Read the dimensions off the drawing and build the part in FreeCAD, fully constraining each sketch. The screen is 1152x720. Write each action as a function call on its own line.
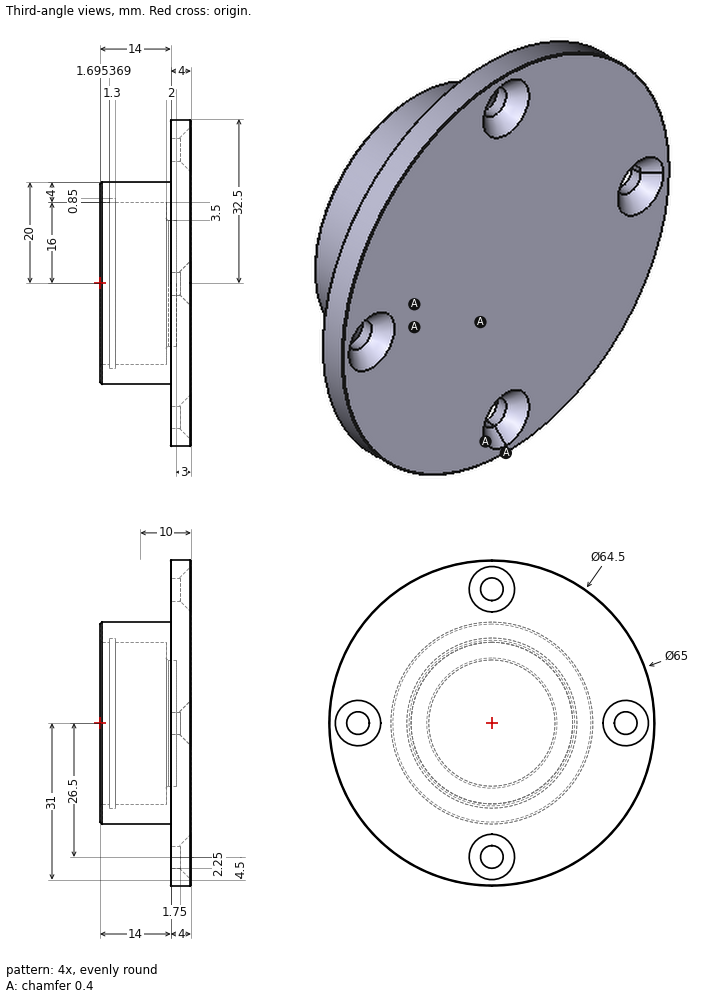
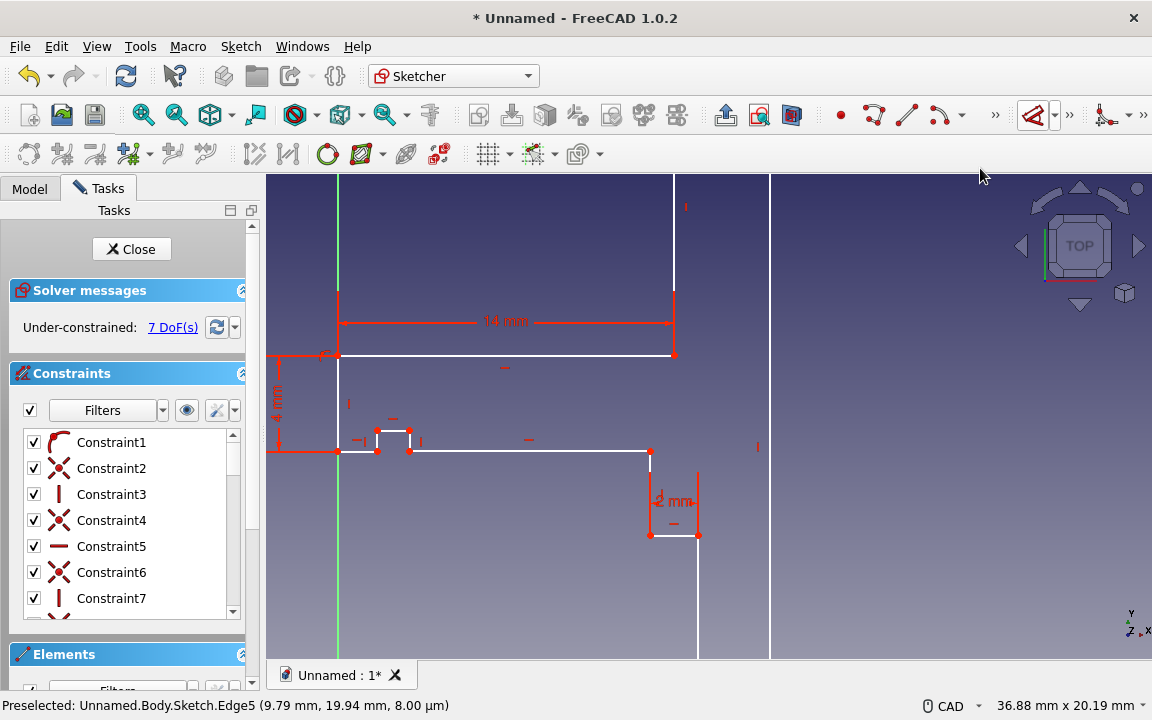
scroll(387, 431, up, 2)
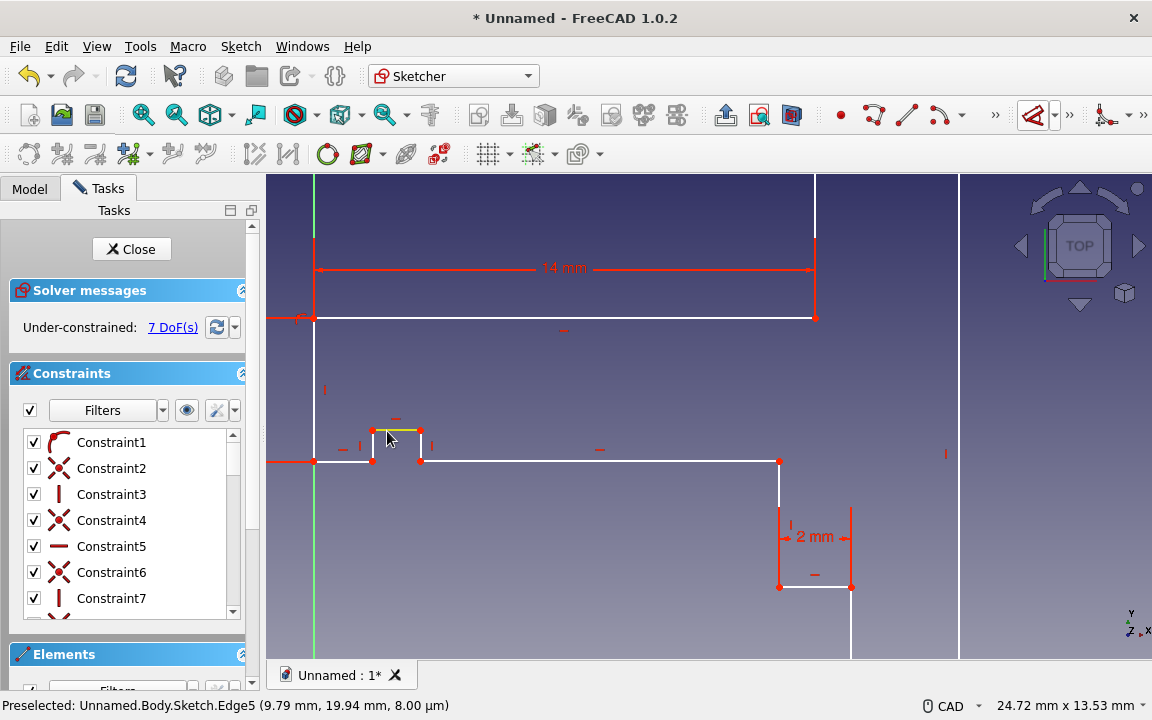
click(387, 430)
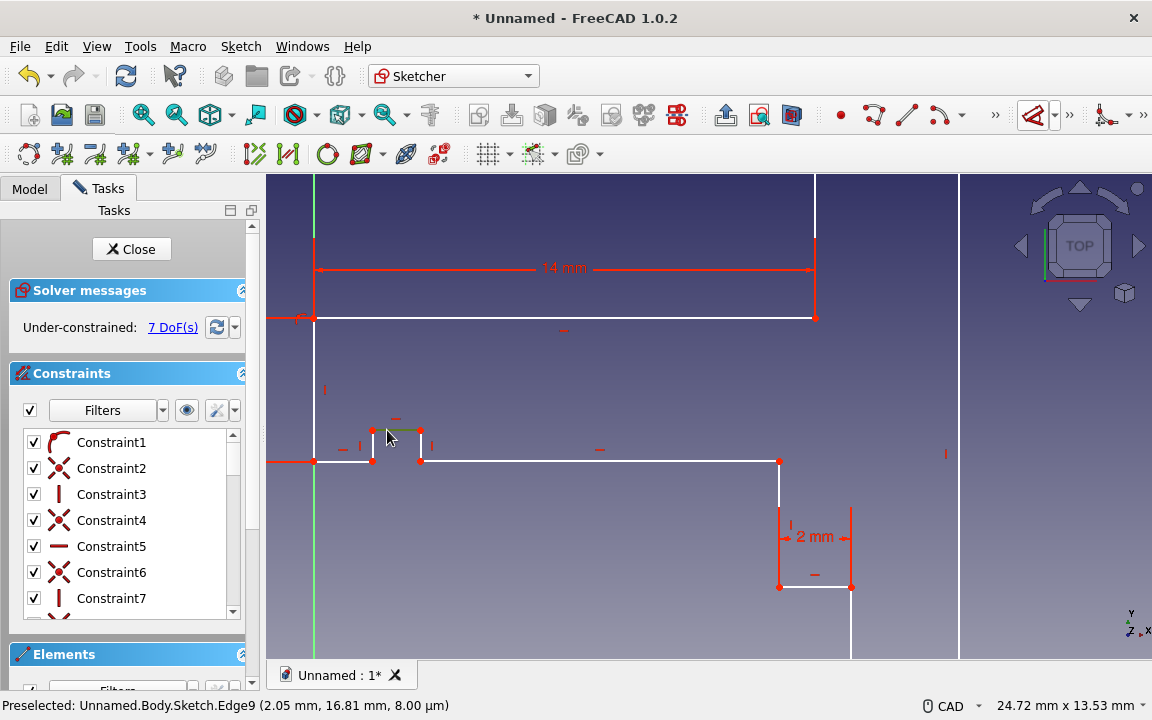
click(1054, 116)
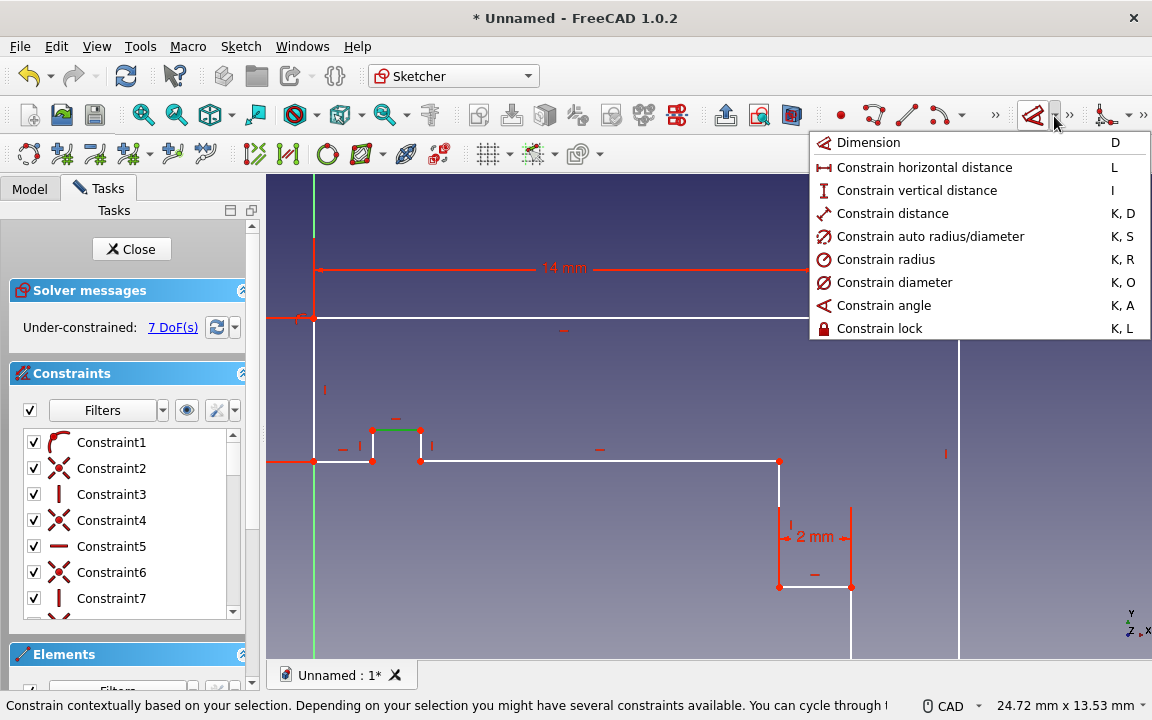
click(980, 168)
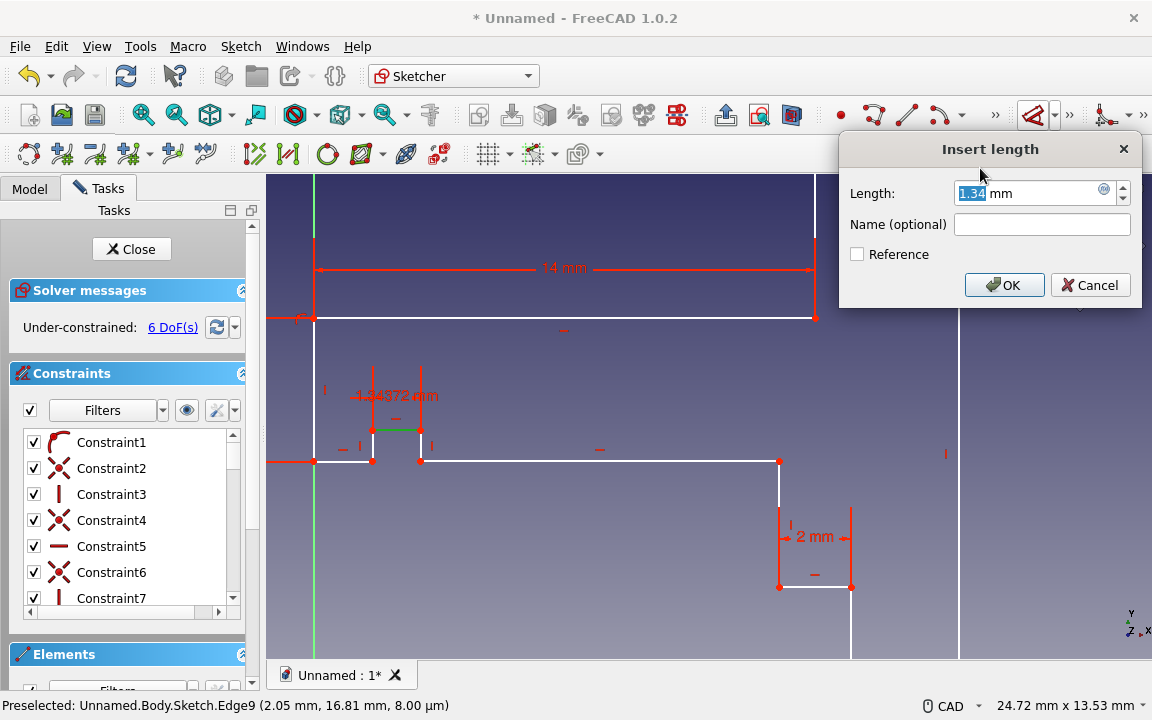
text(1.3)
key(Return)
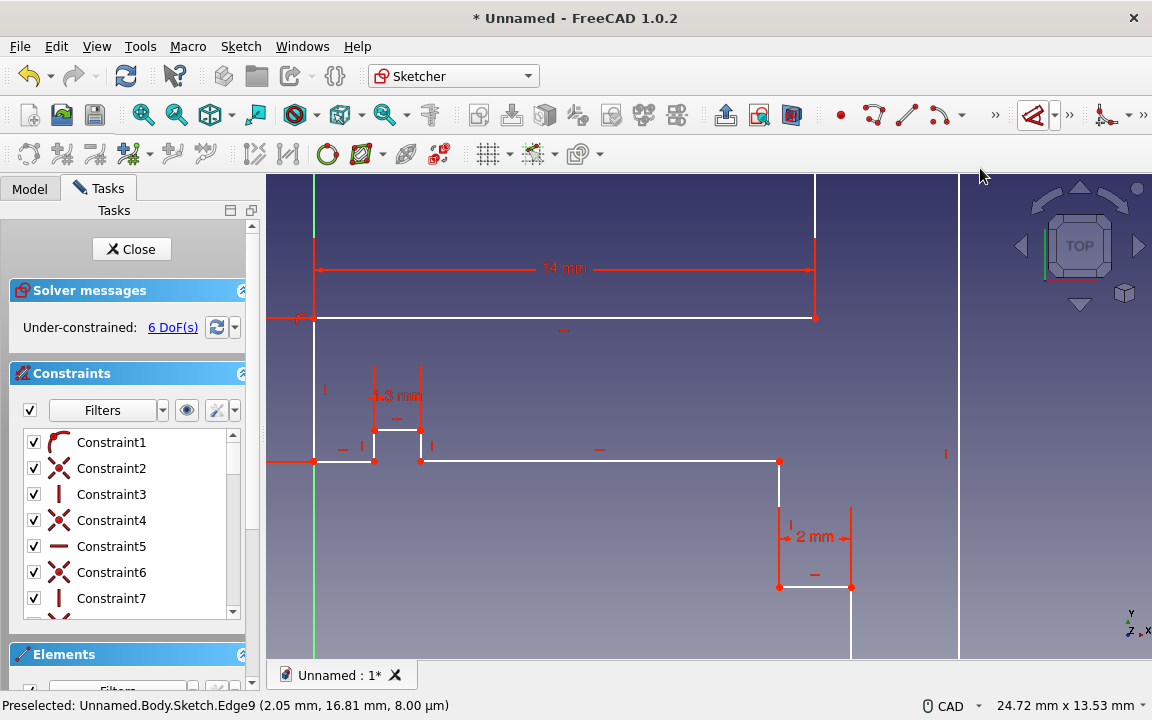
click(779, 499)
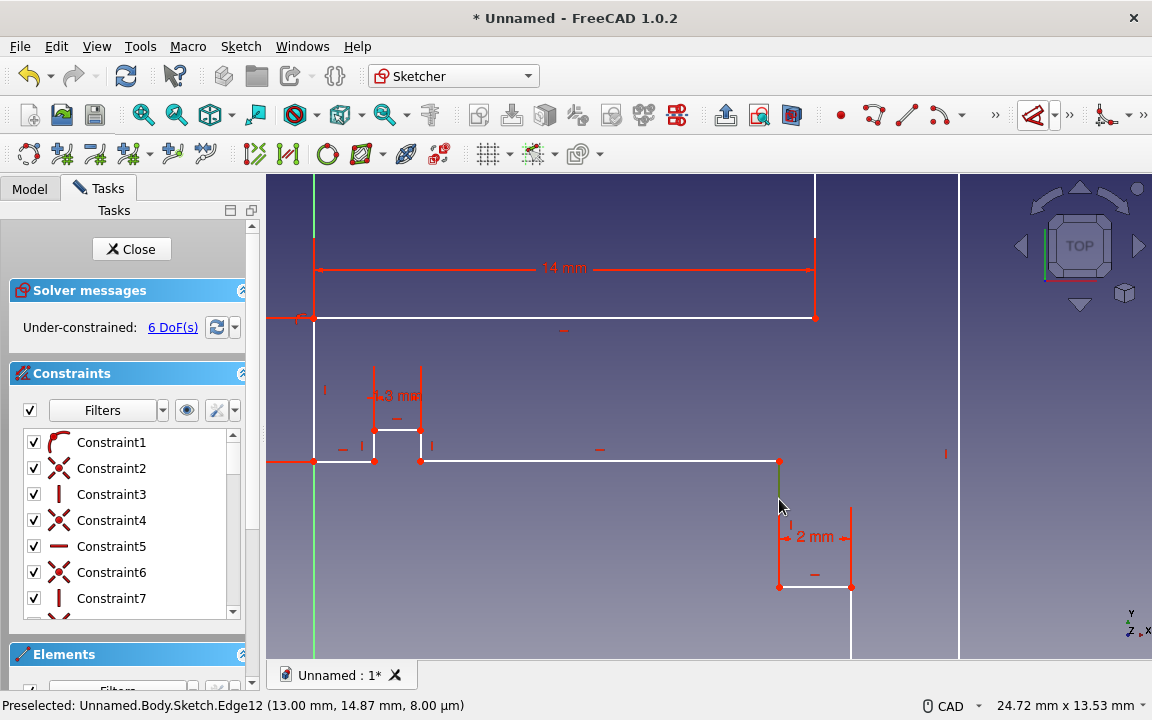
click(1054, 116)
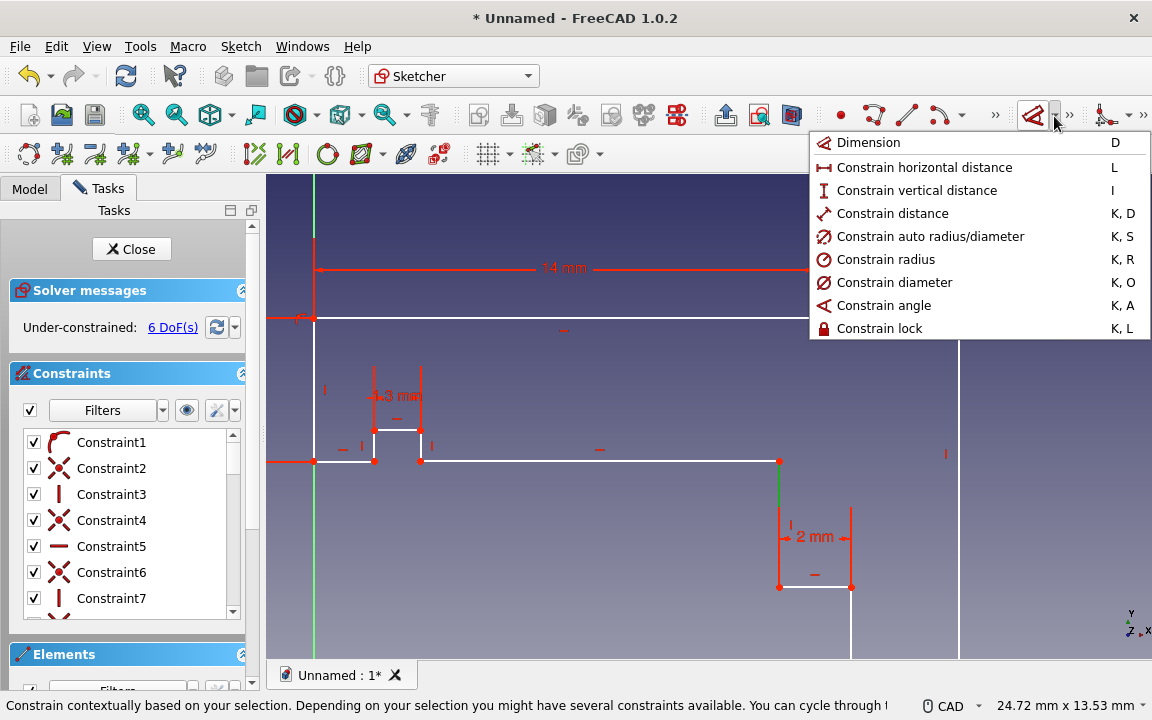
click(980, 190)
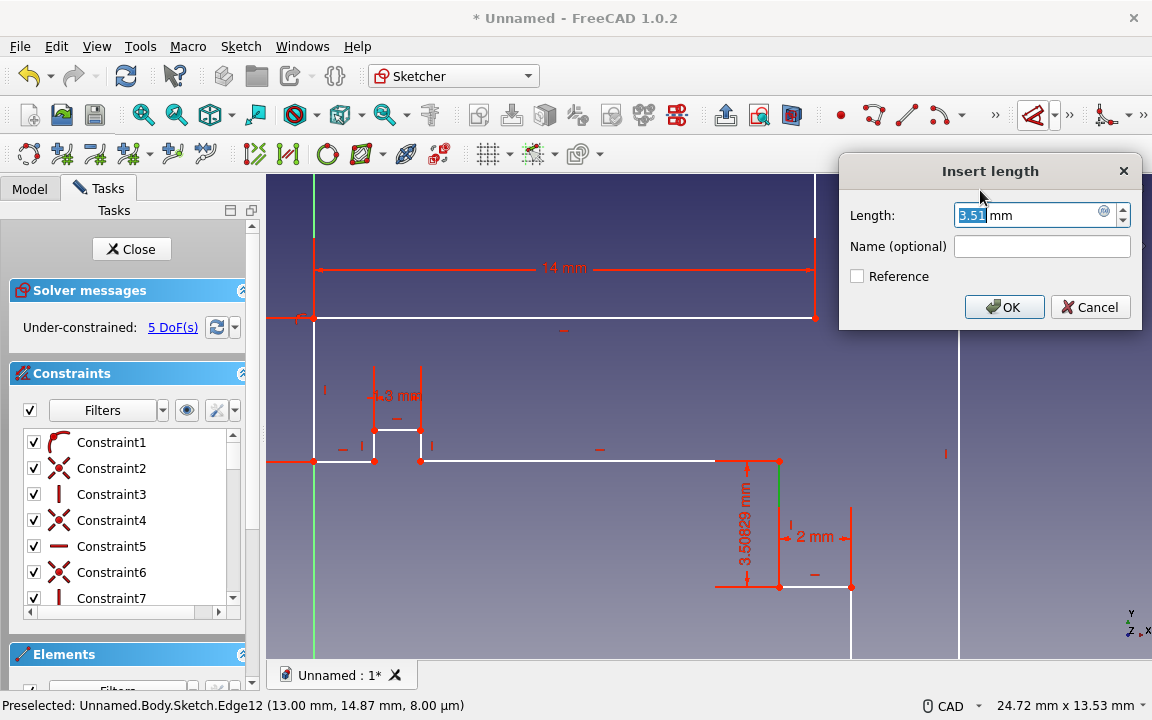
text(3.5)
key(Return)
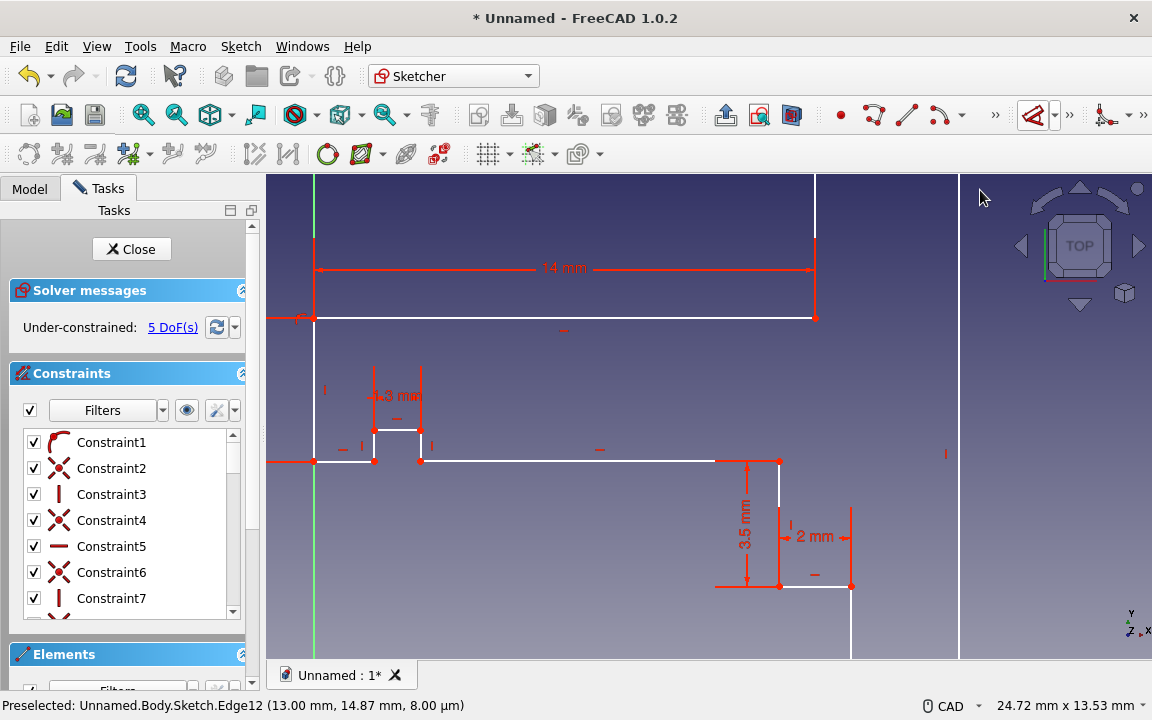
scroll(642, 405, down, 7)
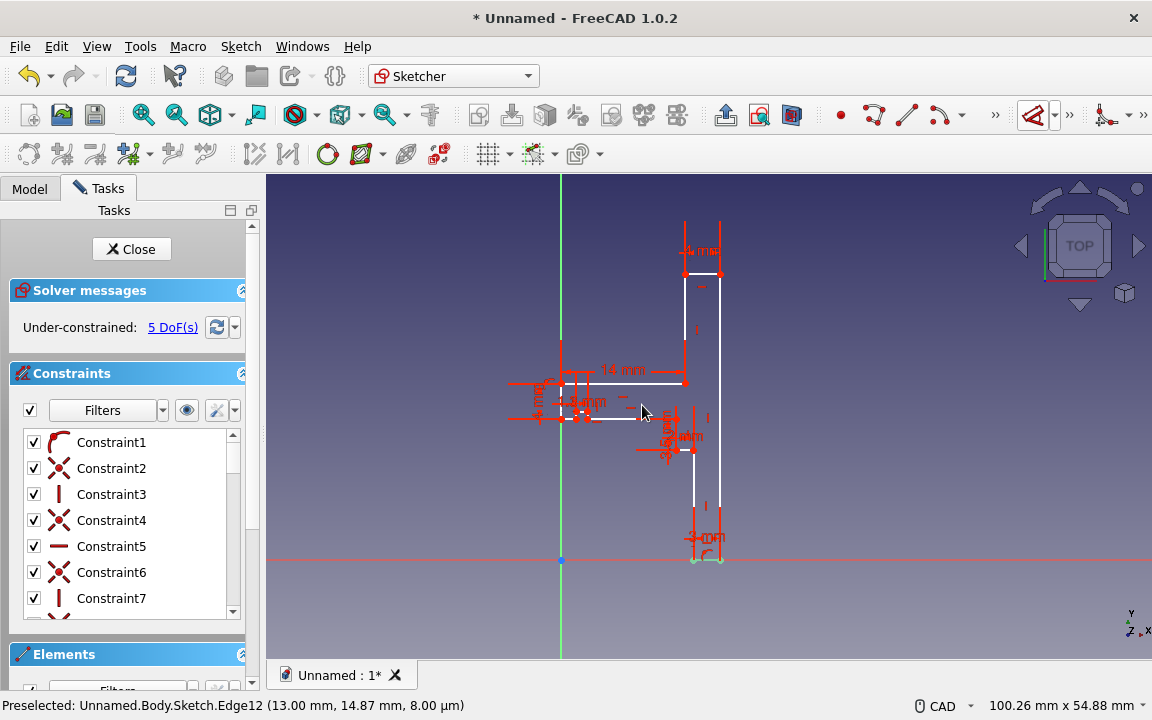
click(685, 384)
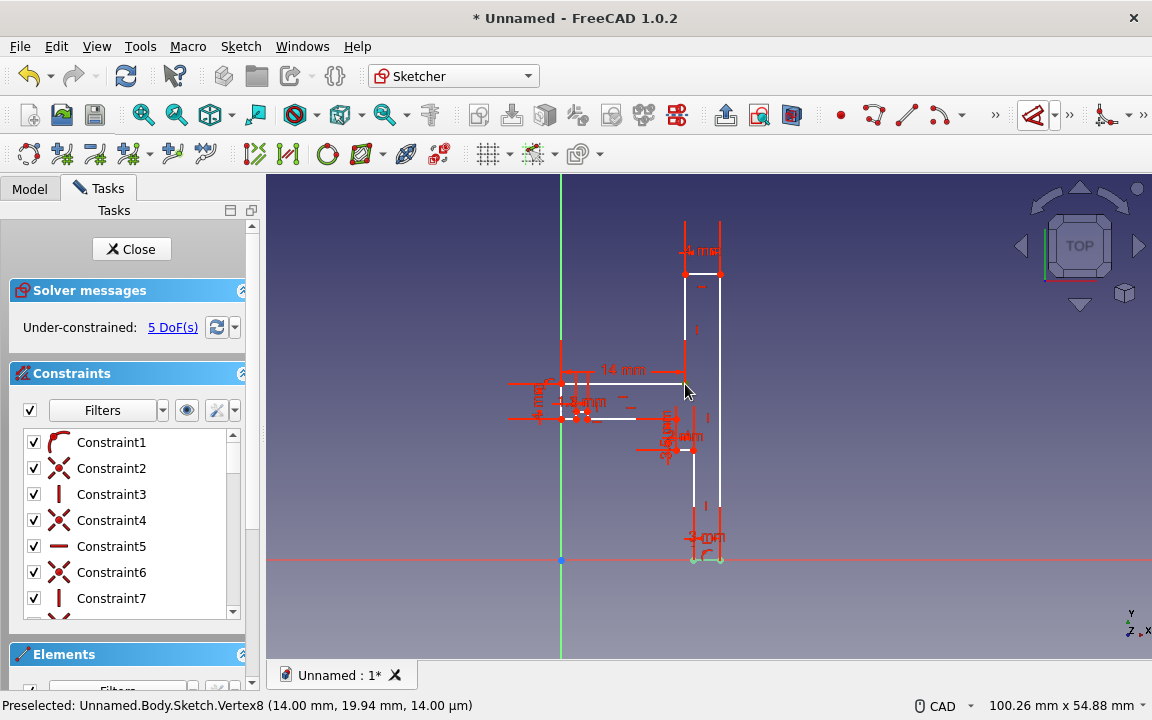
click(1054, 116)